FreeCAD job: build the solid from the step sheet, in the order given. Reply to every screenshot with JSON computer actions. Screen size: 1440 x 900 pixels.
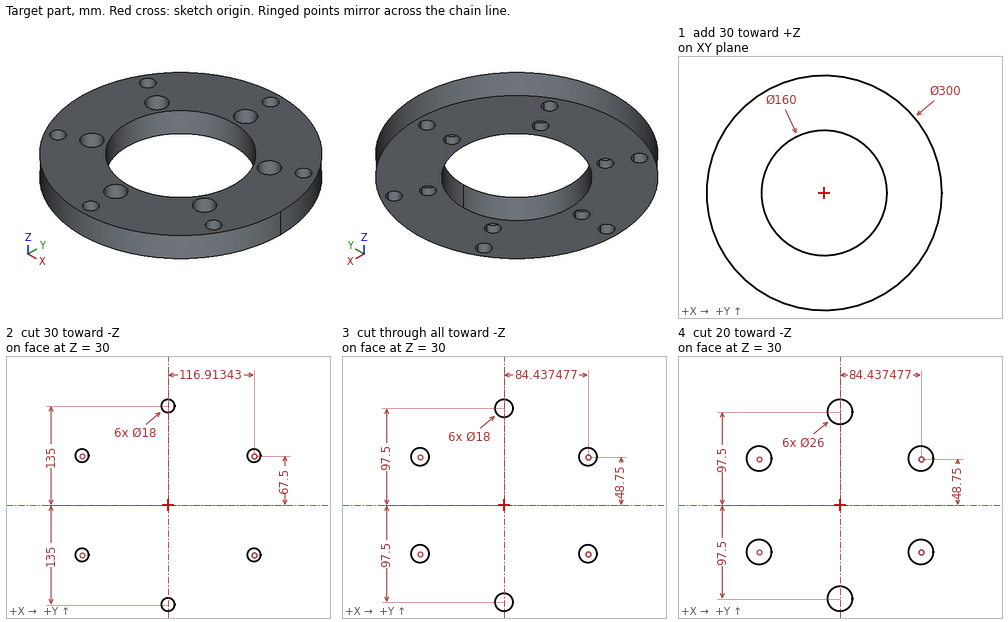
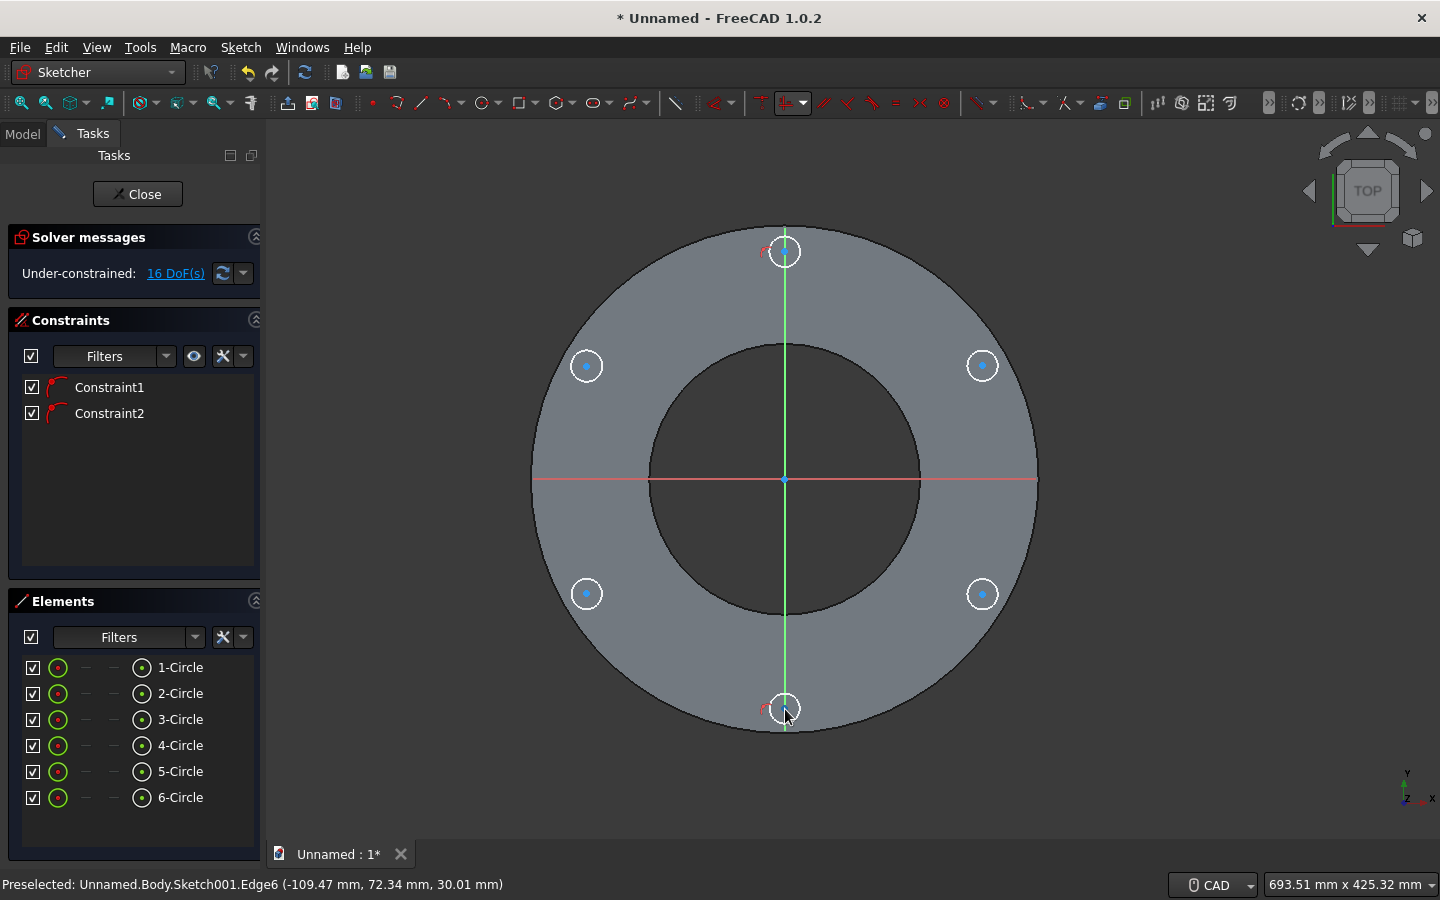
{"action": "scroll", "coordinate": [795, 241], "scroll_direction": "up", "scroll_amount": 2}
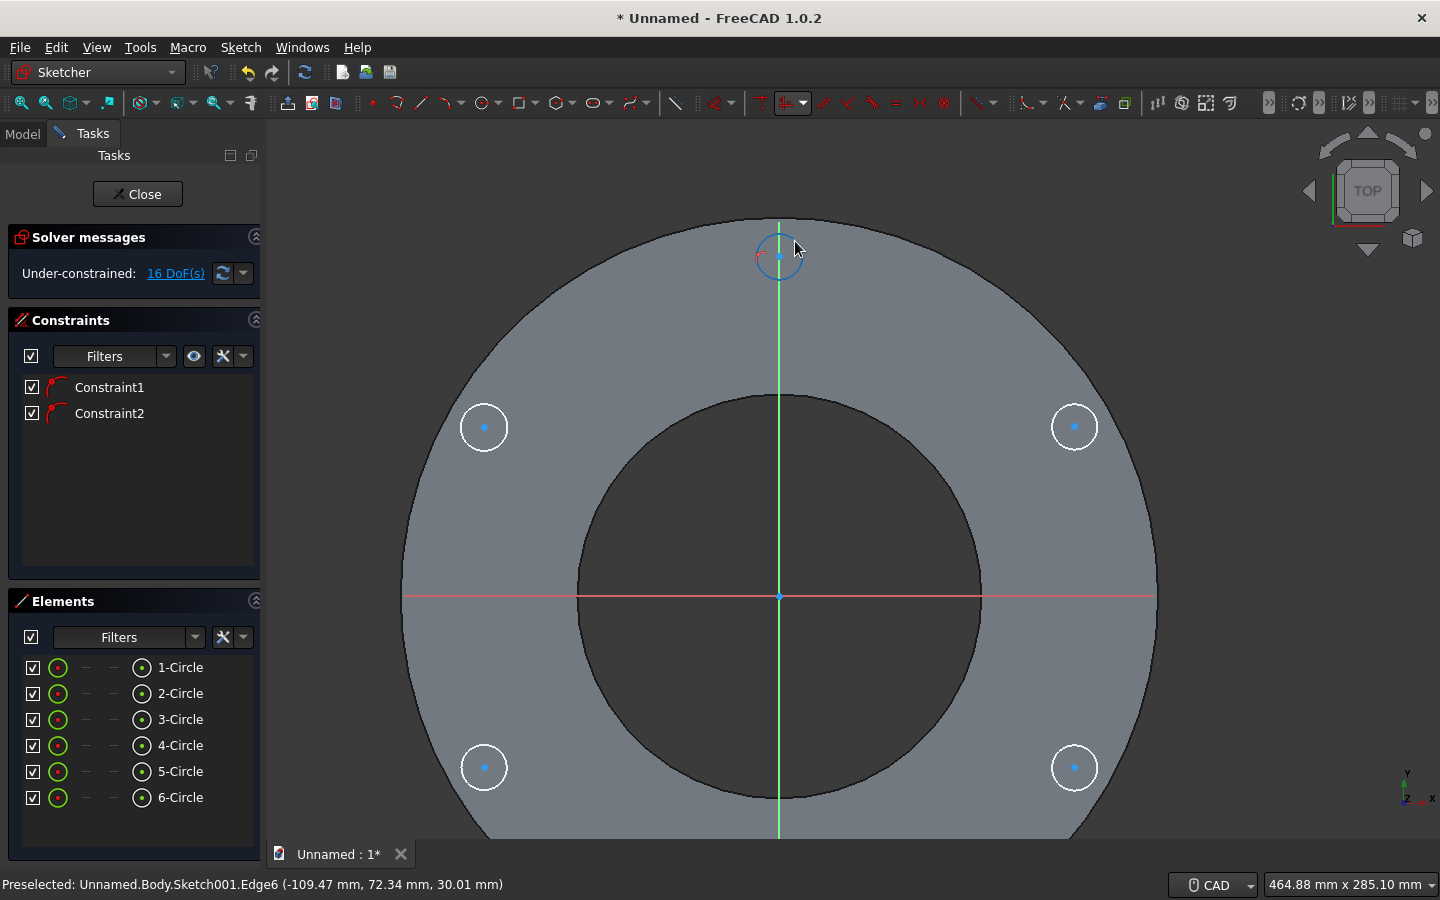
{"action": "left_click", "coordinate": [795, 241]}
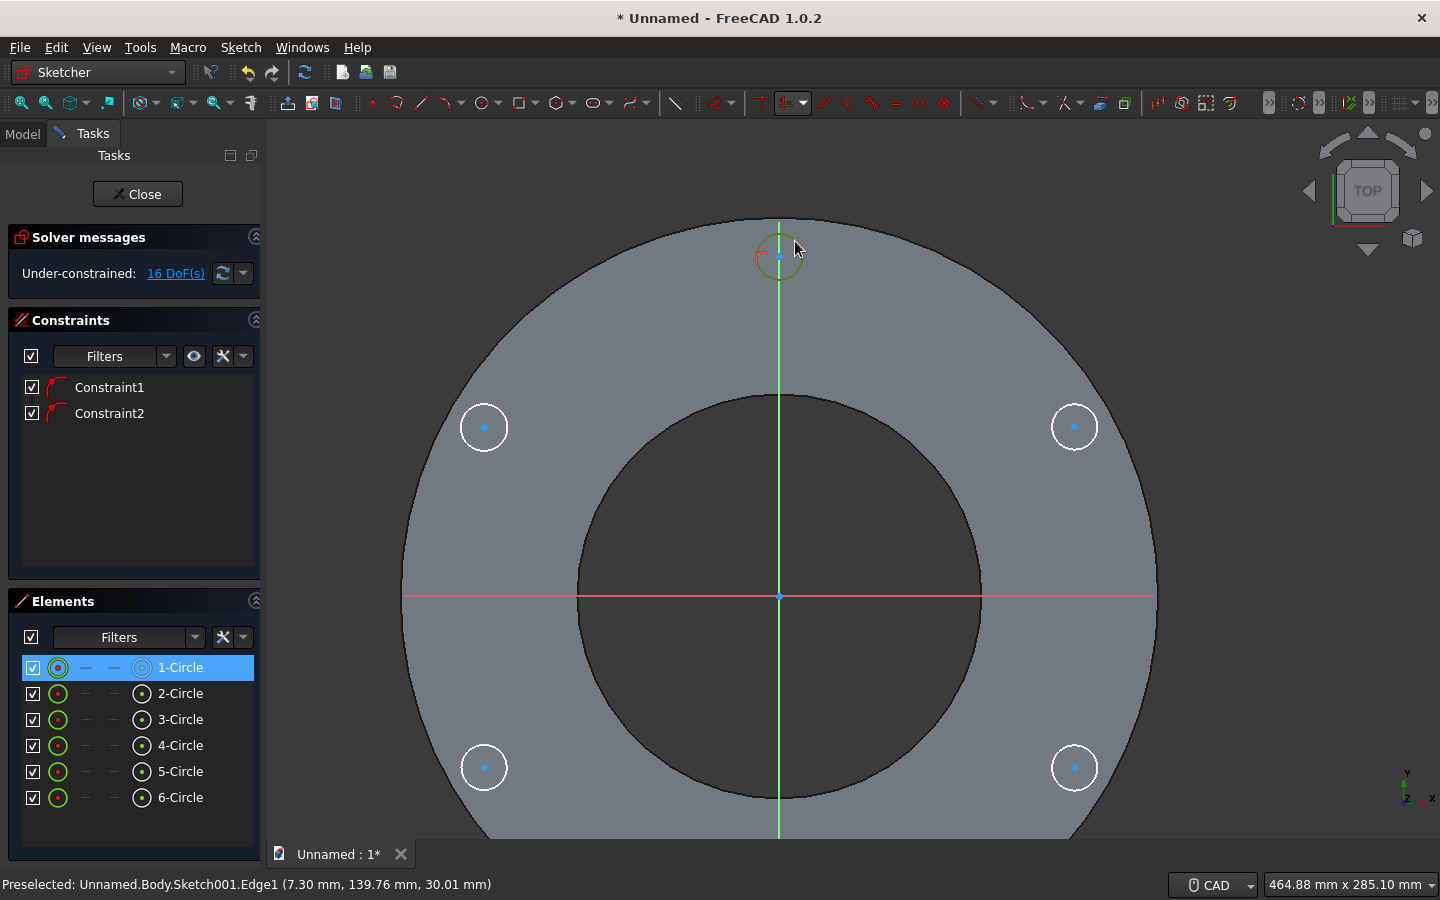
{"action": "left_click", "coordinate": [1091, 411]}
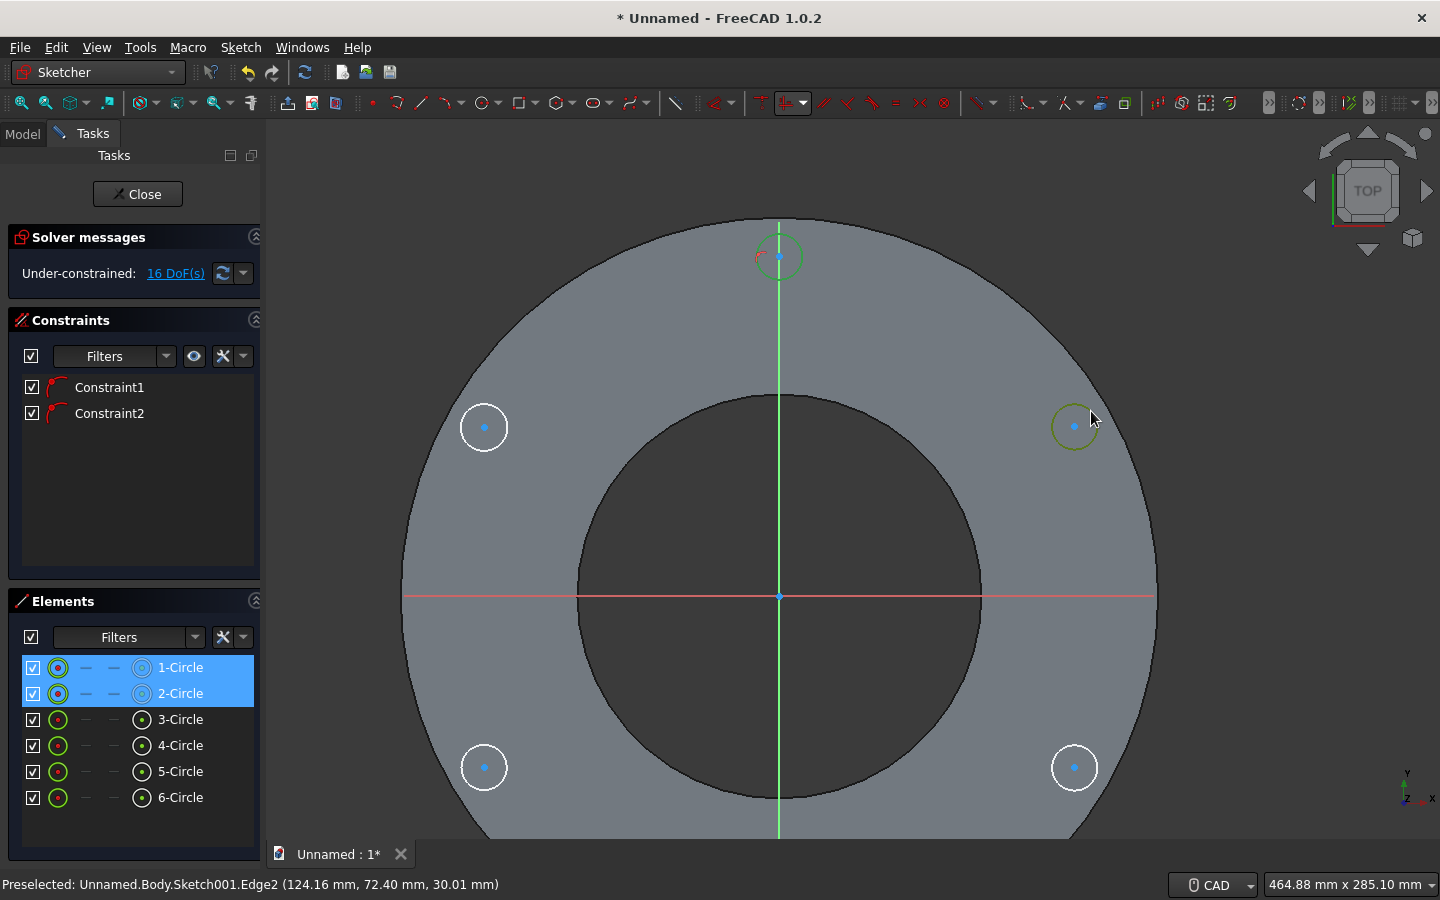
{"action": "left_click", "coordinate": [1091, 752]}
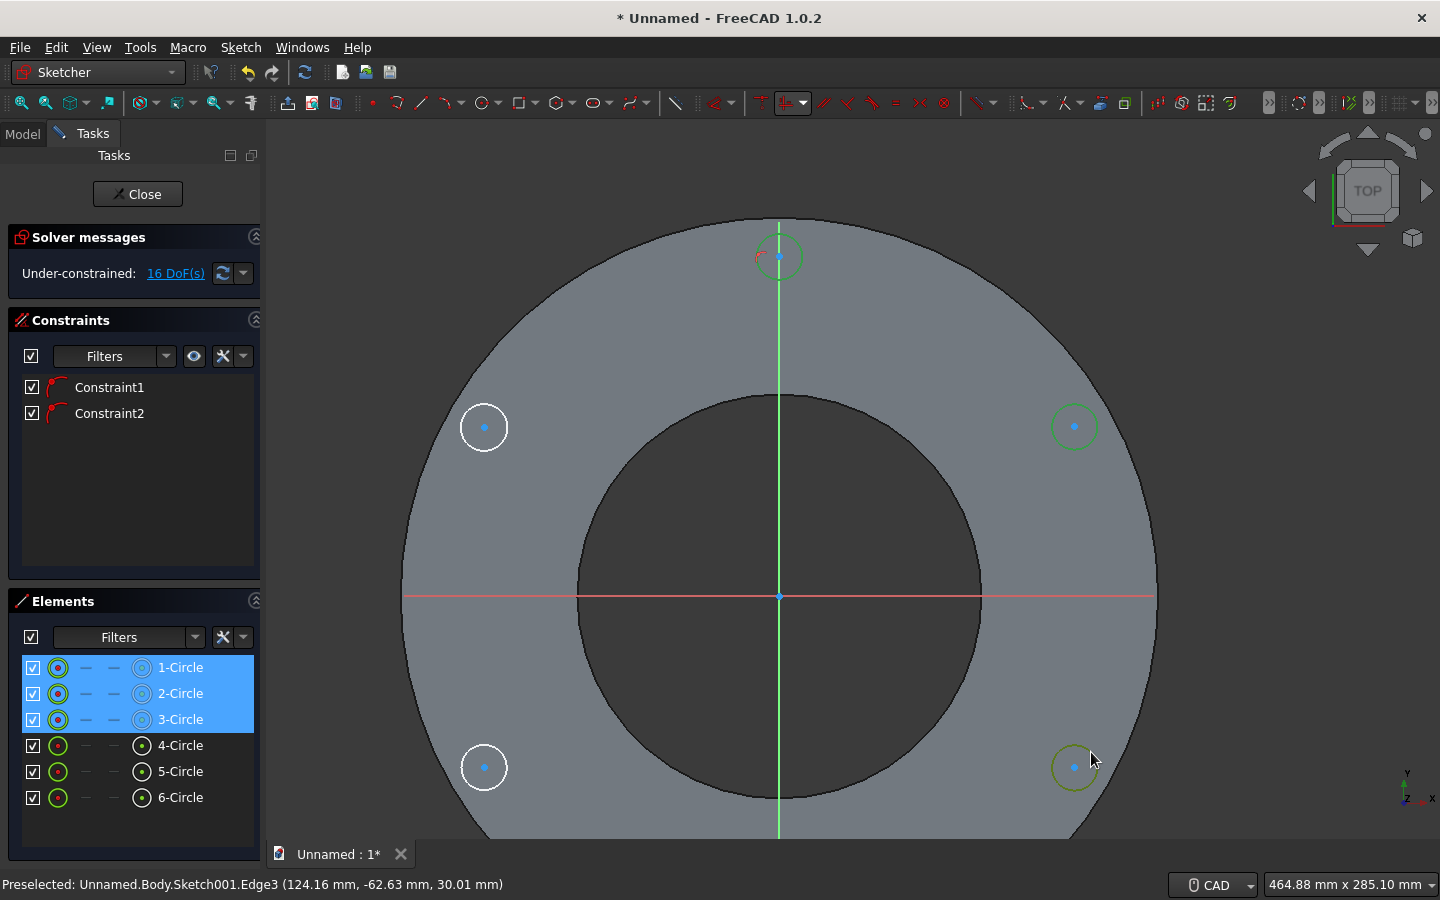
{"action": "scroll", "coordinate": [795, 240], "scroll_direction": "down", "scroll_amount": 2}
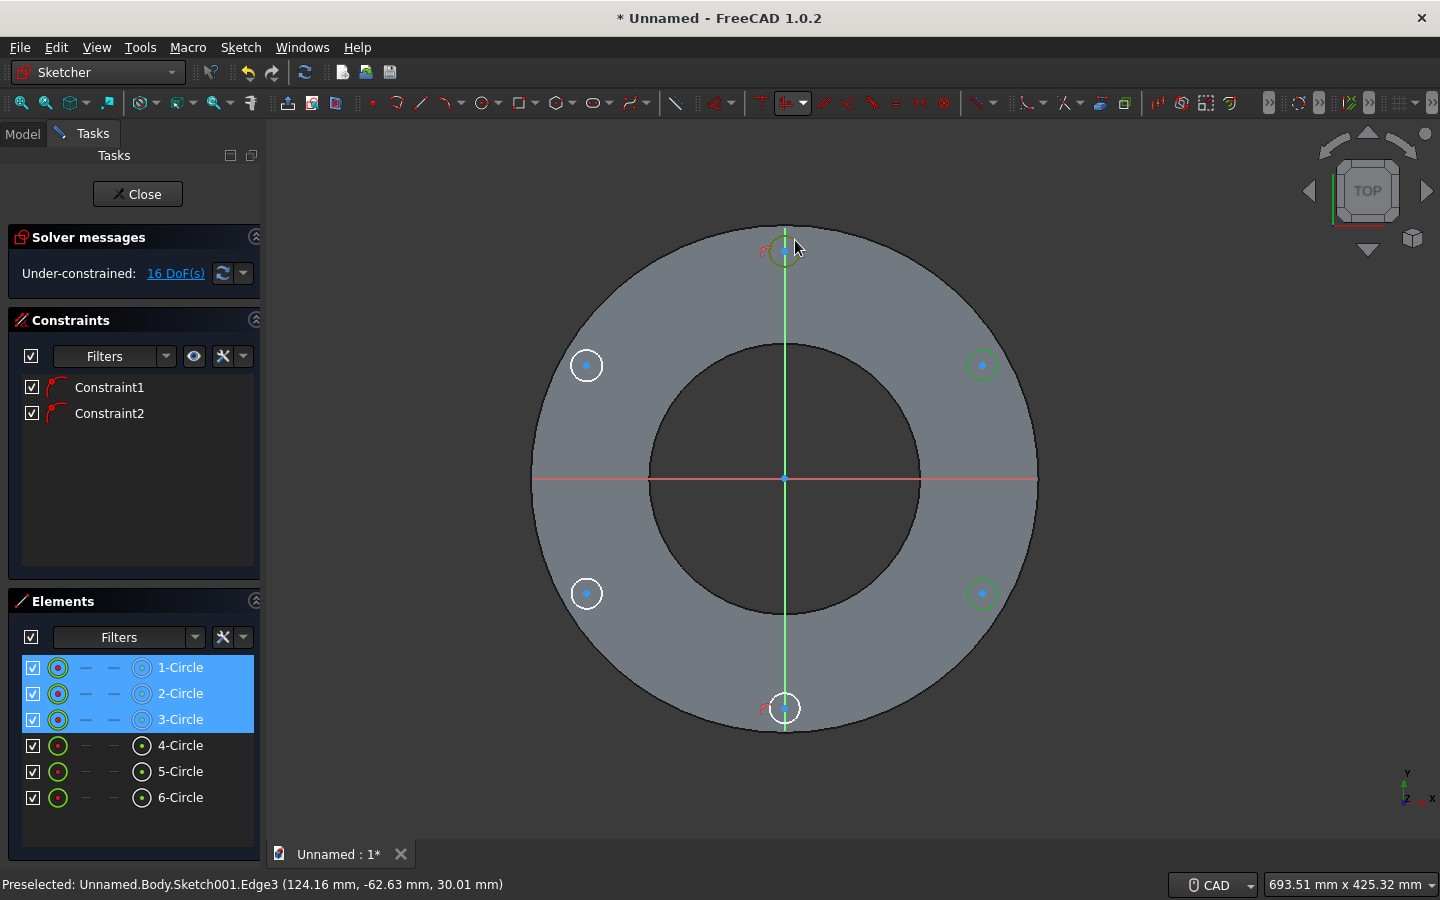
{"action": "scroll", "coordinate": [795, 698], "scroll_direction": "up", "scroll_amount": 2}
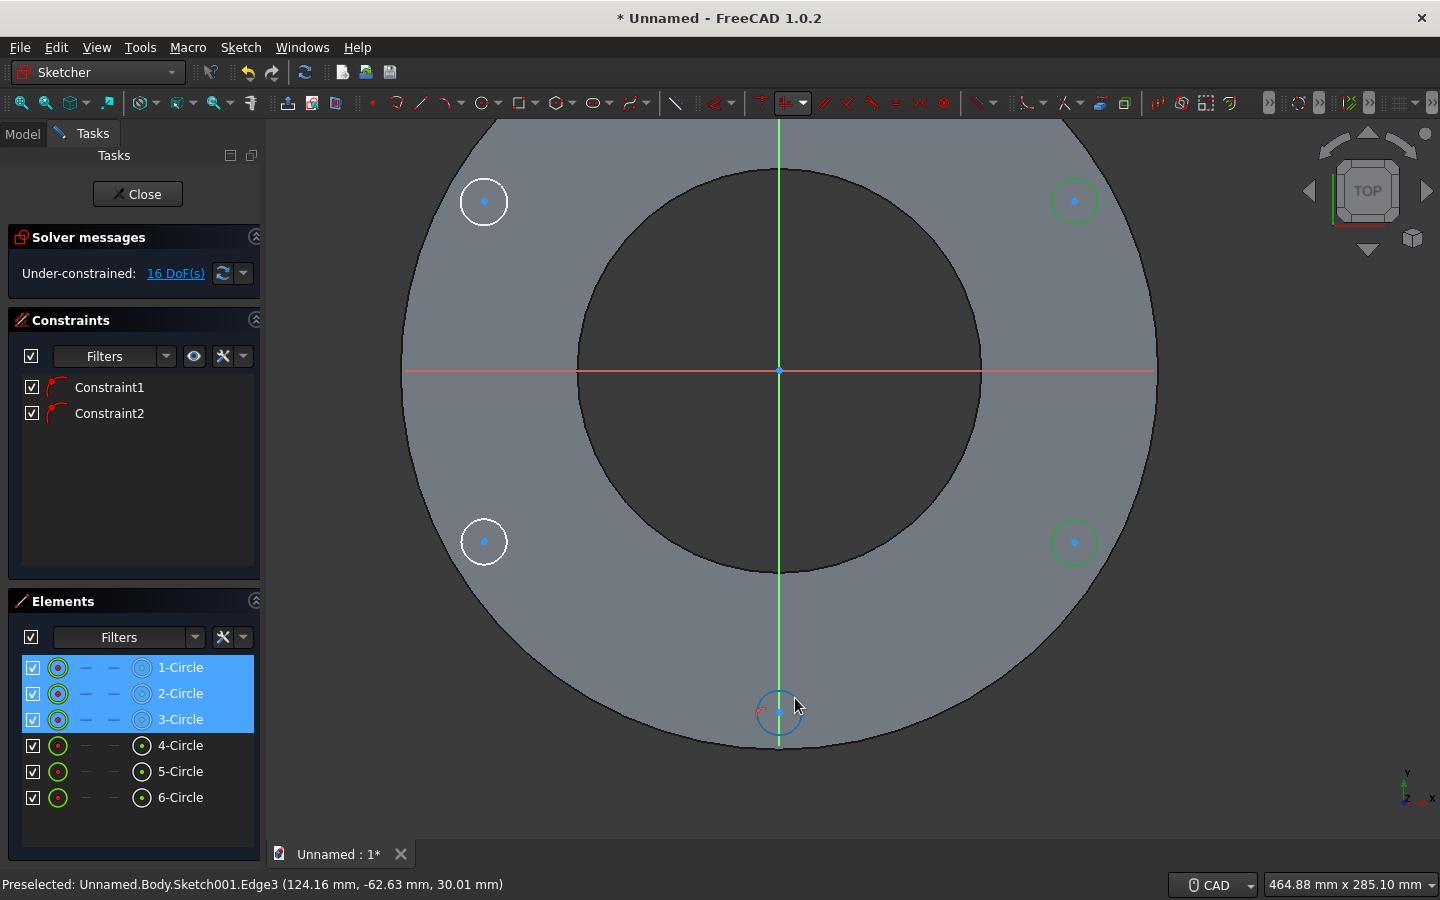
{"action": "left_click", "coordinate": [795, 697]}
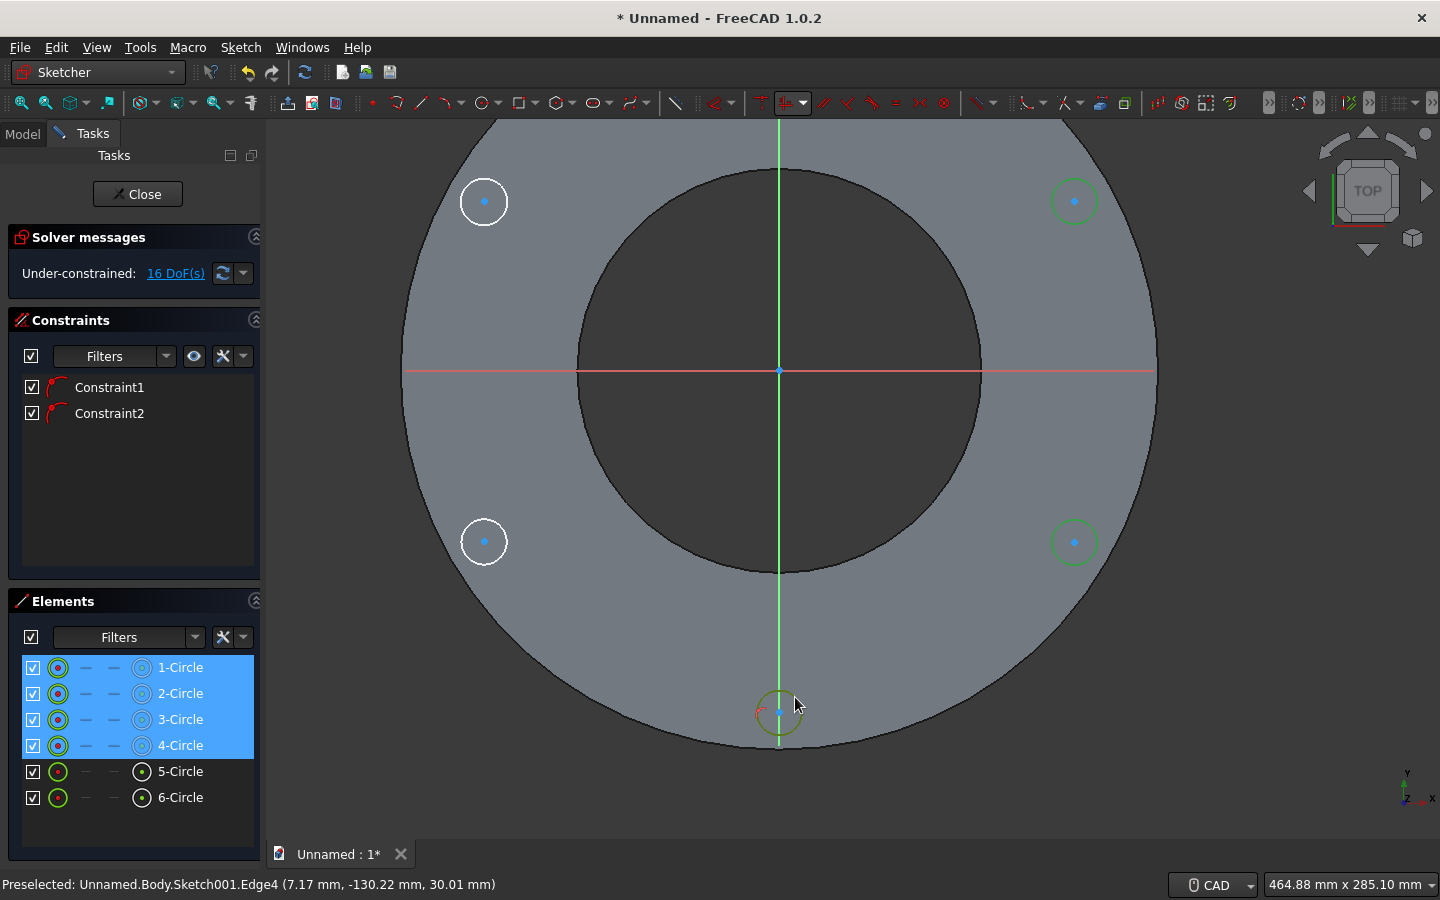
{"action": "left_click", "coordinate": [500, 526]}